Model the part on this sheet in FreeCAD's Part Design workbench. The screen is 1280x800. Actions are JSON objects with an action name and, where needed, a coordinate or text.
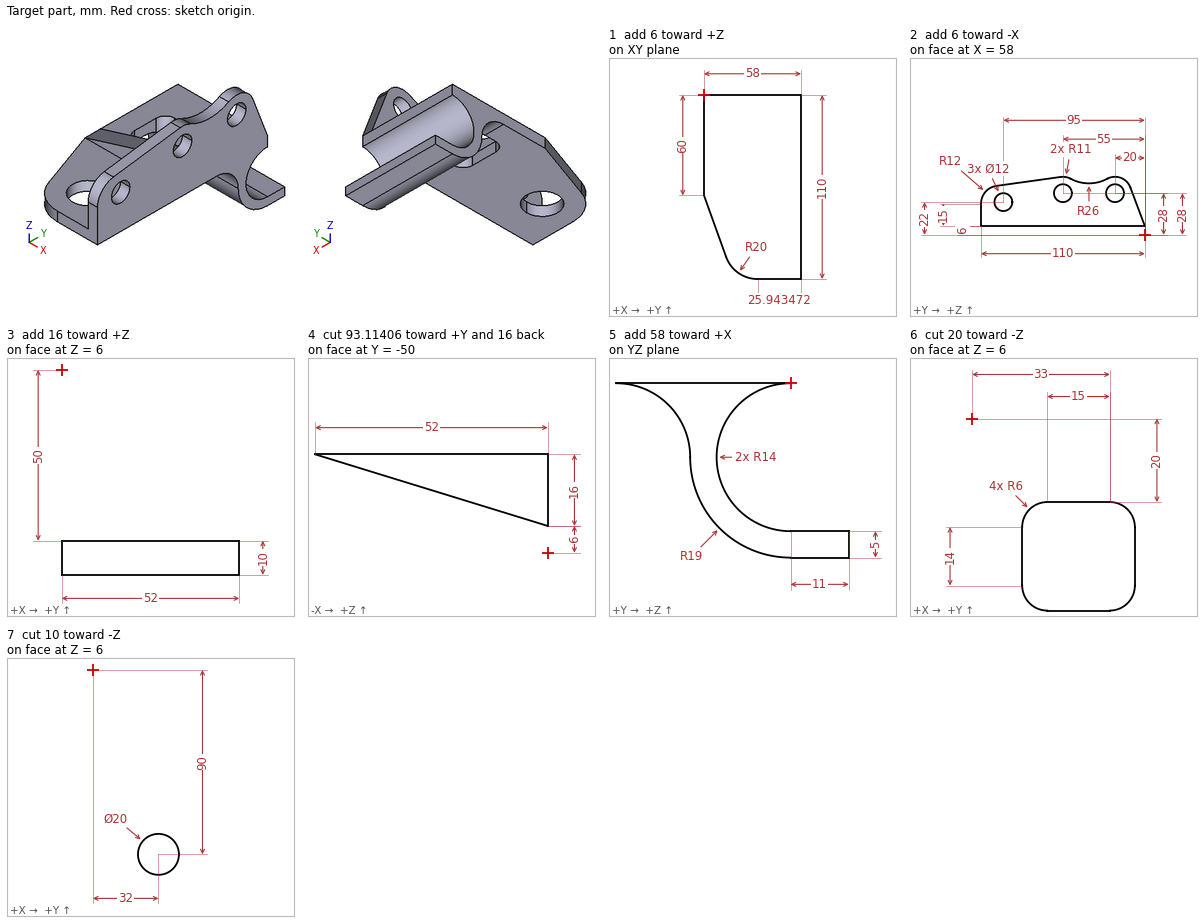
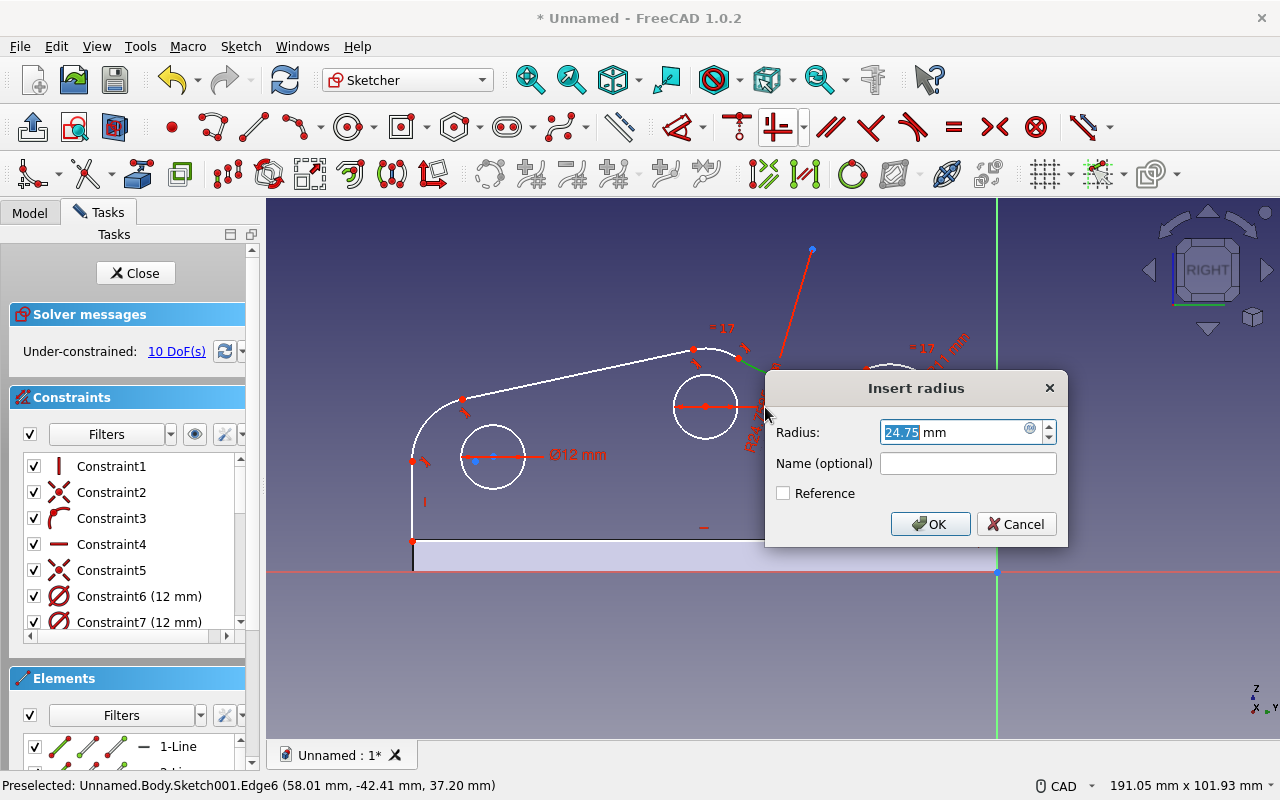
{"action": "type", "text": "26"}
{"action": "key", "text": "Return"}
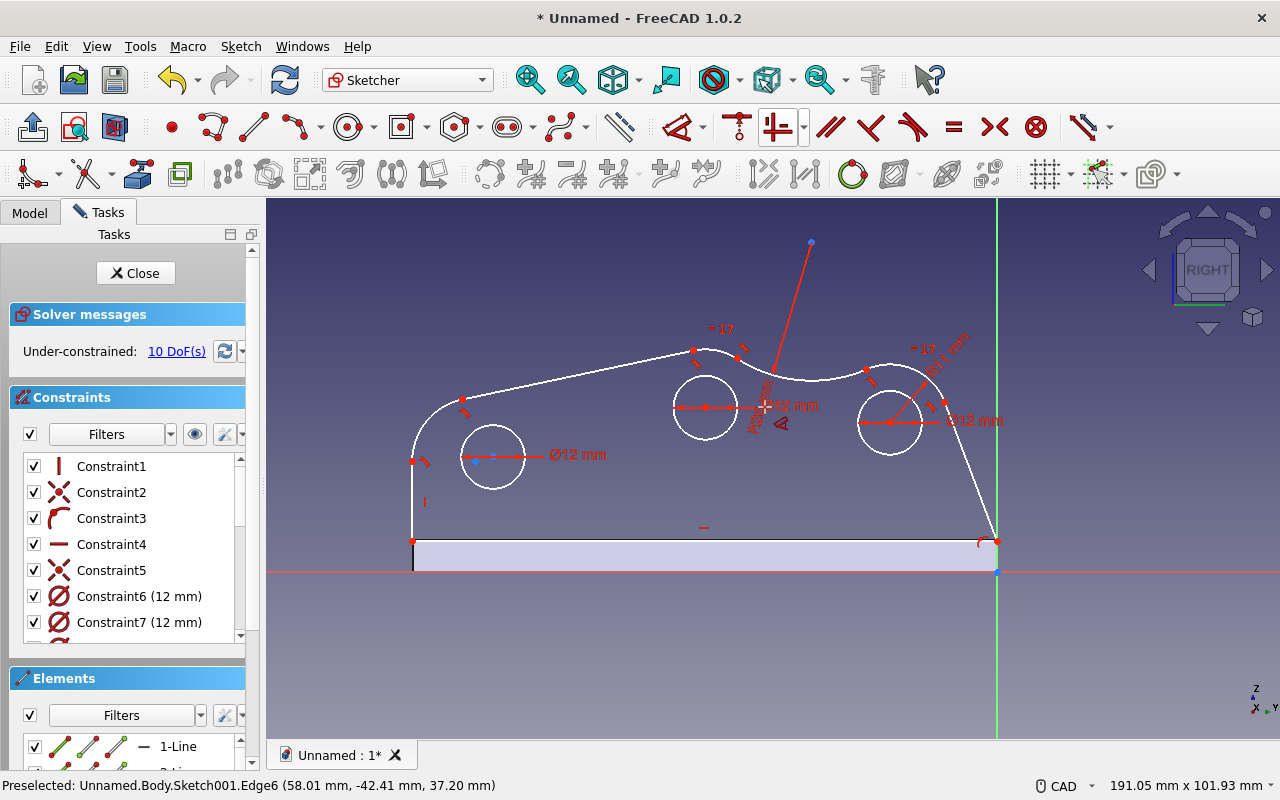
{"action": "left_click", "coordinate": [439, 410]}
{"action": "left_click", "coordinate": [420, 384]}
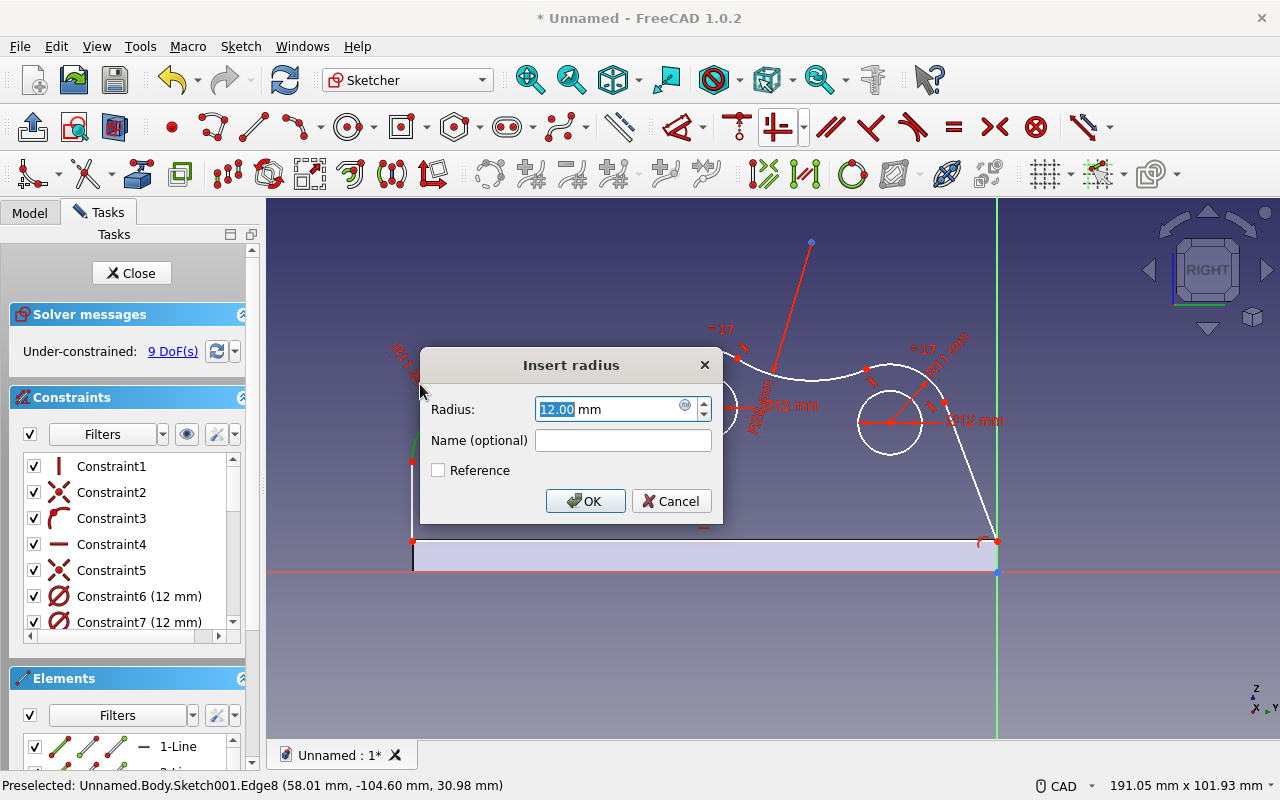
{"action": "type", "text": "12"}
{"action": "key", "text": "Return"}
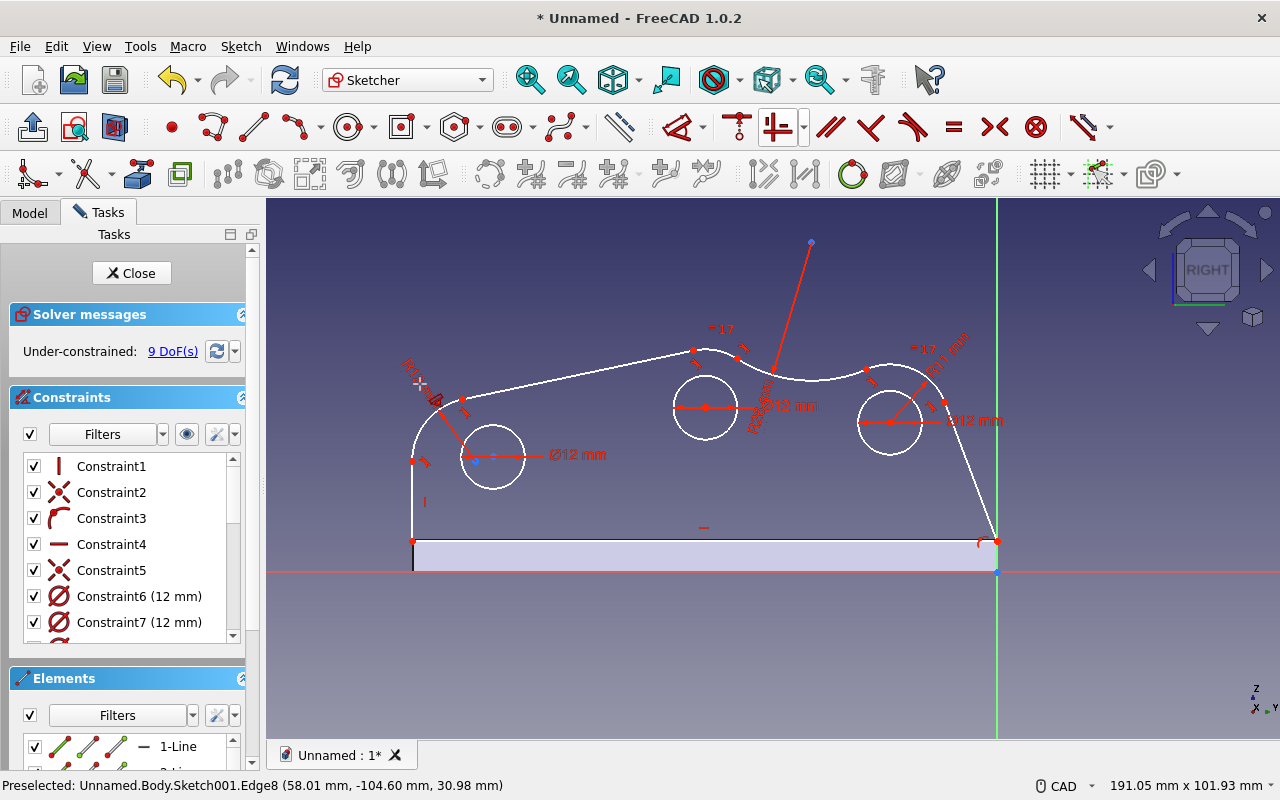
{"action": "left_click", "coordinate": [412, 486]}
{"action": "left_click", "coordinate": [378, 501]}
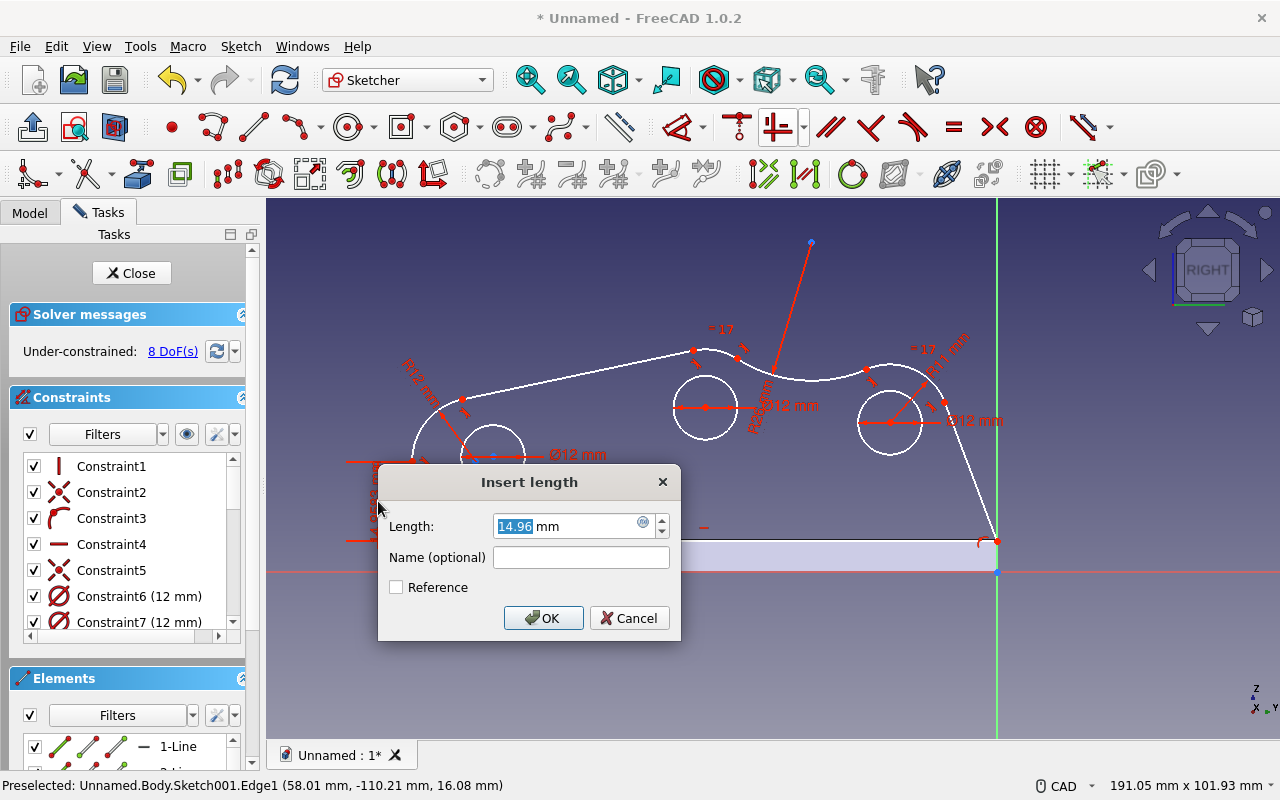
{"action": "type", "text": "15"}
{"action": "key", "text": "Return"}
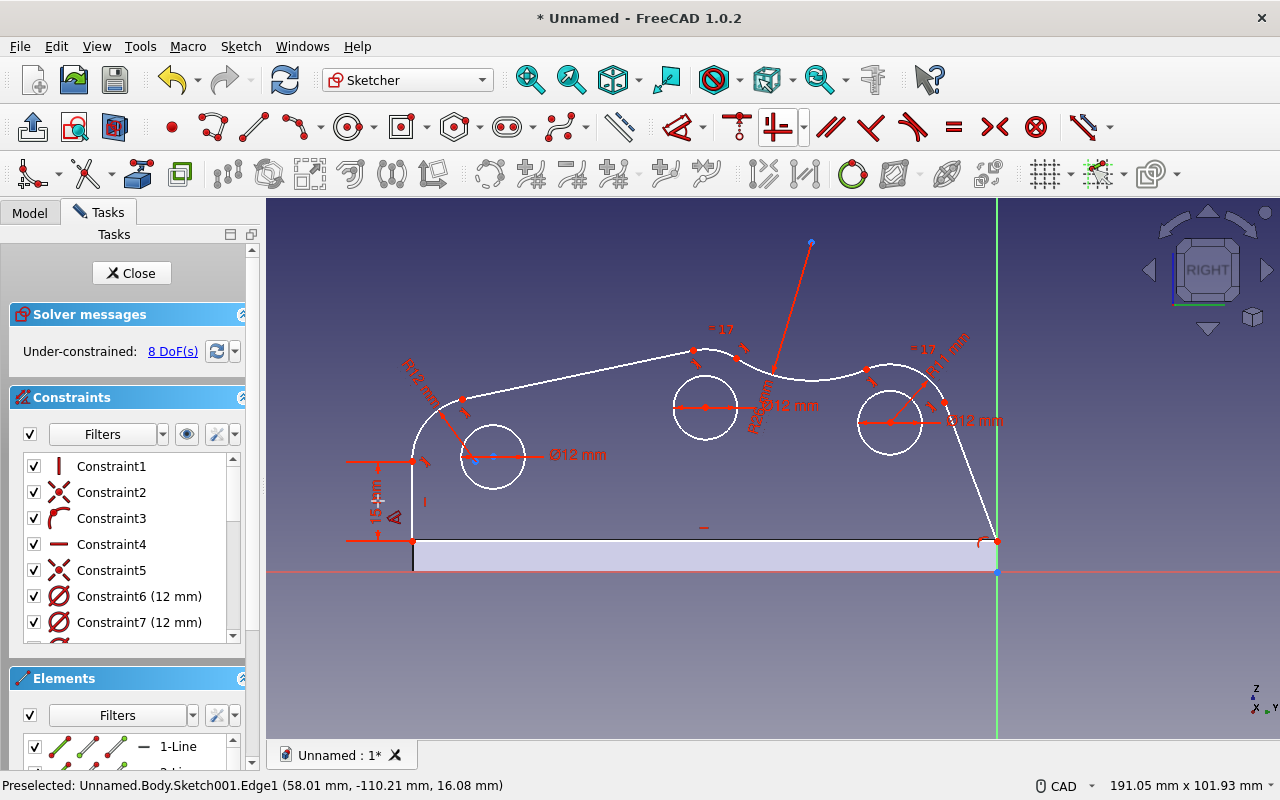
{"action": "scroll", "coordinate": [412, 541], "scroll_direction": "up", "scroll_amount": 2}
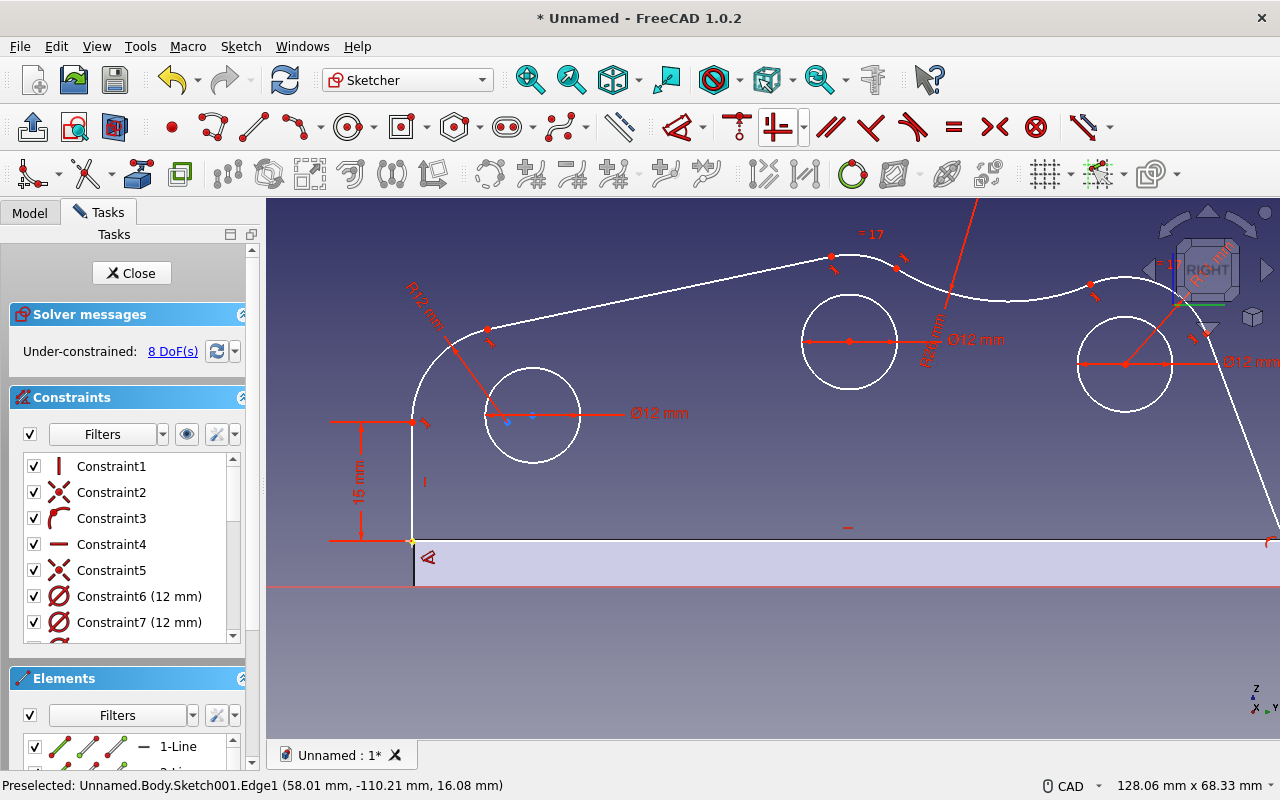
{"action": "left_click", "coordinate": [412, 541]}
{"action": "left_click", "coordinate": [378, 564]}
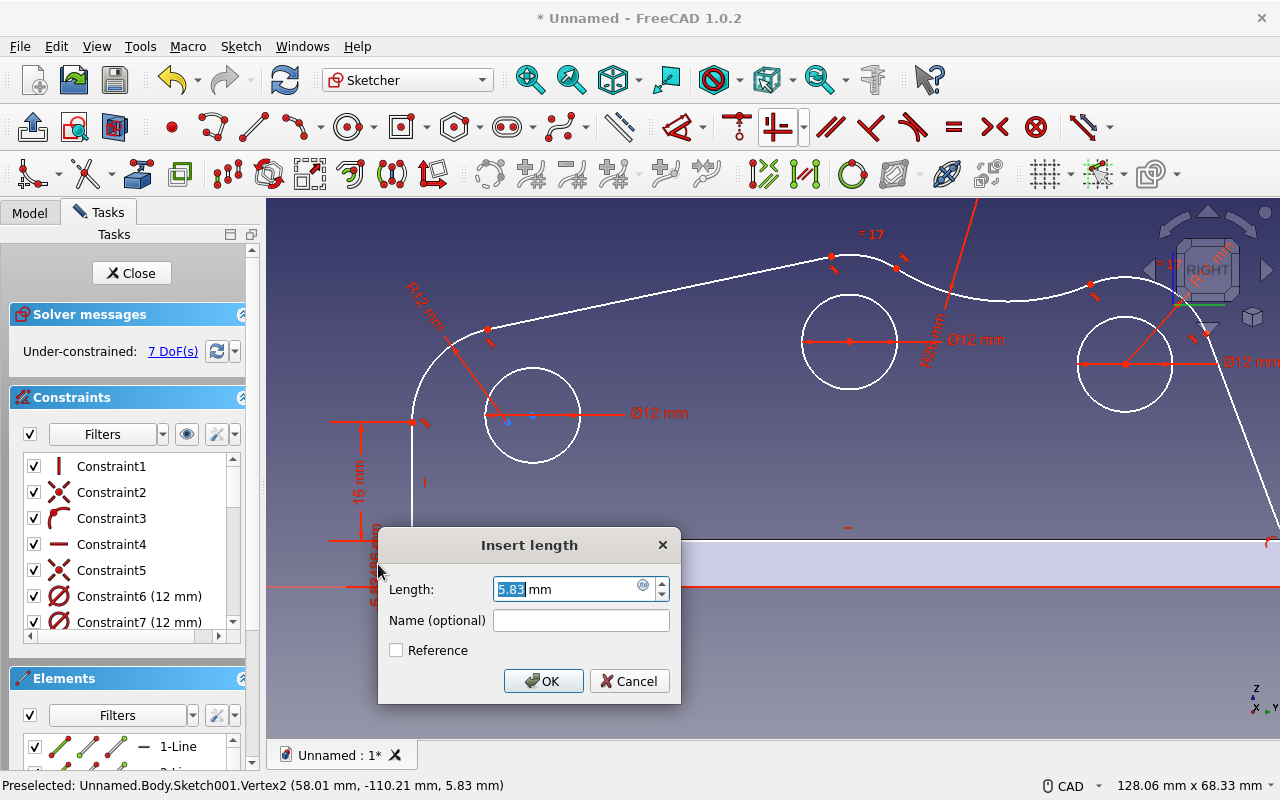
{"action": "type", "text": "6"}
{"action": "key", "text": "Return"}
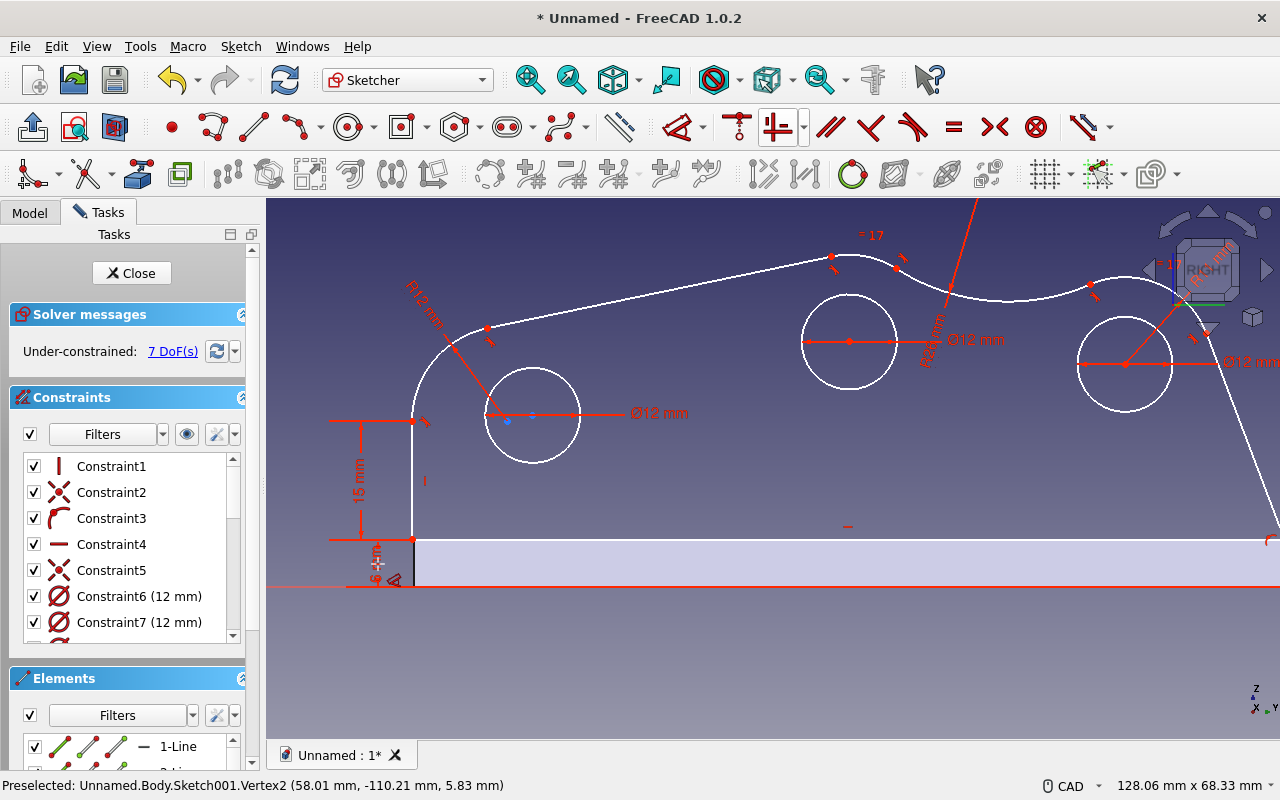
{"action": "left_click", "coordinate": [533, 415]}
{"action": "left_click", "coordinate": [824, 621]}